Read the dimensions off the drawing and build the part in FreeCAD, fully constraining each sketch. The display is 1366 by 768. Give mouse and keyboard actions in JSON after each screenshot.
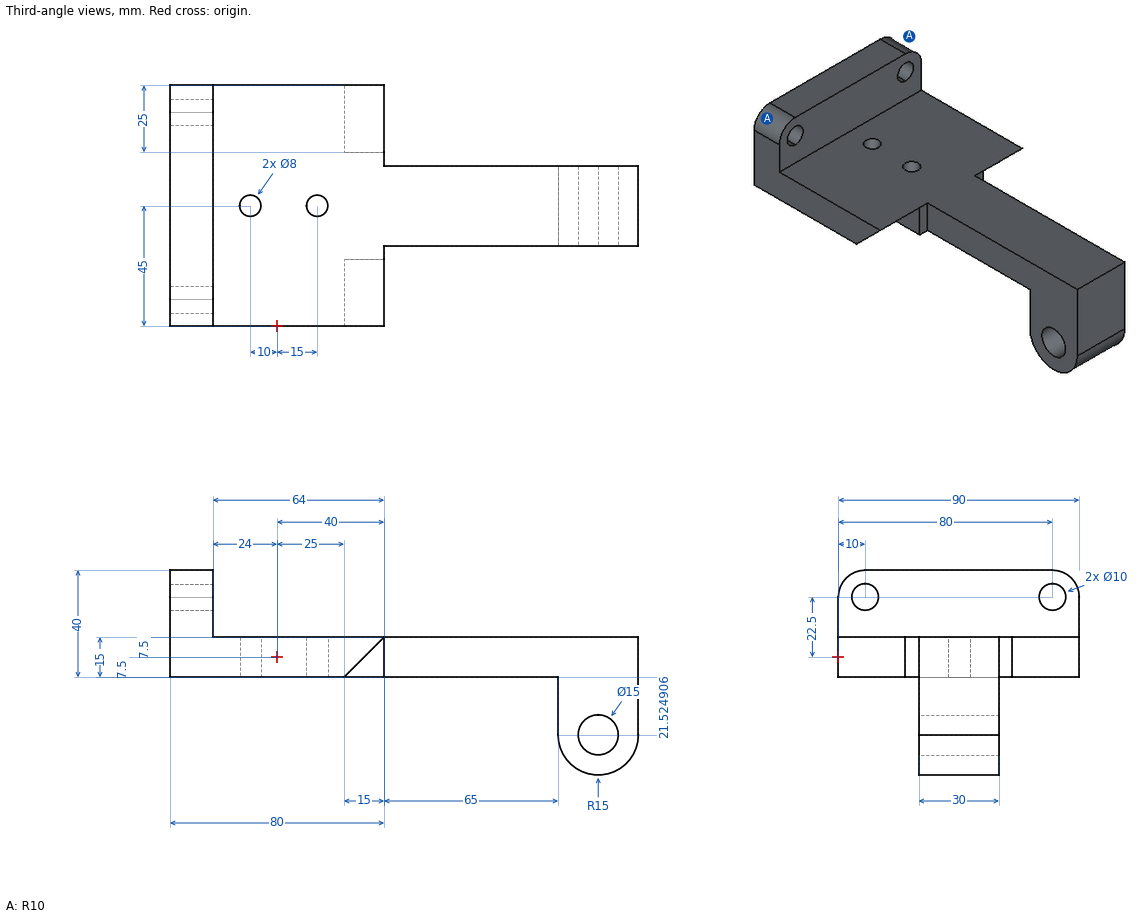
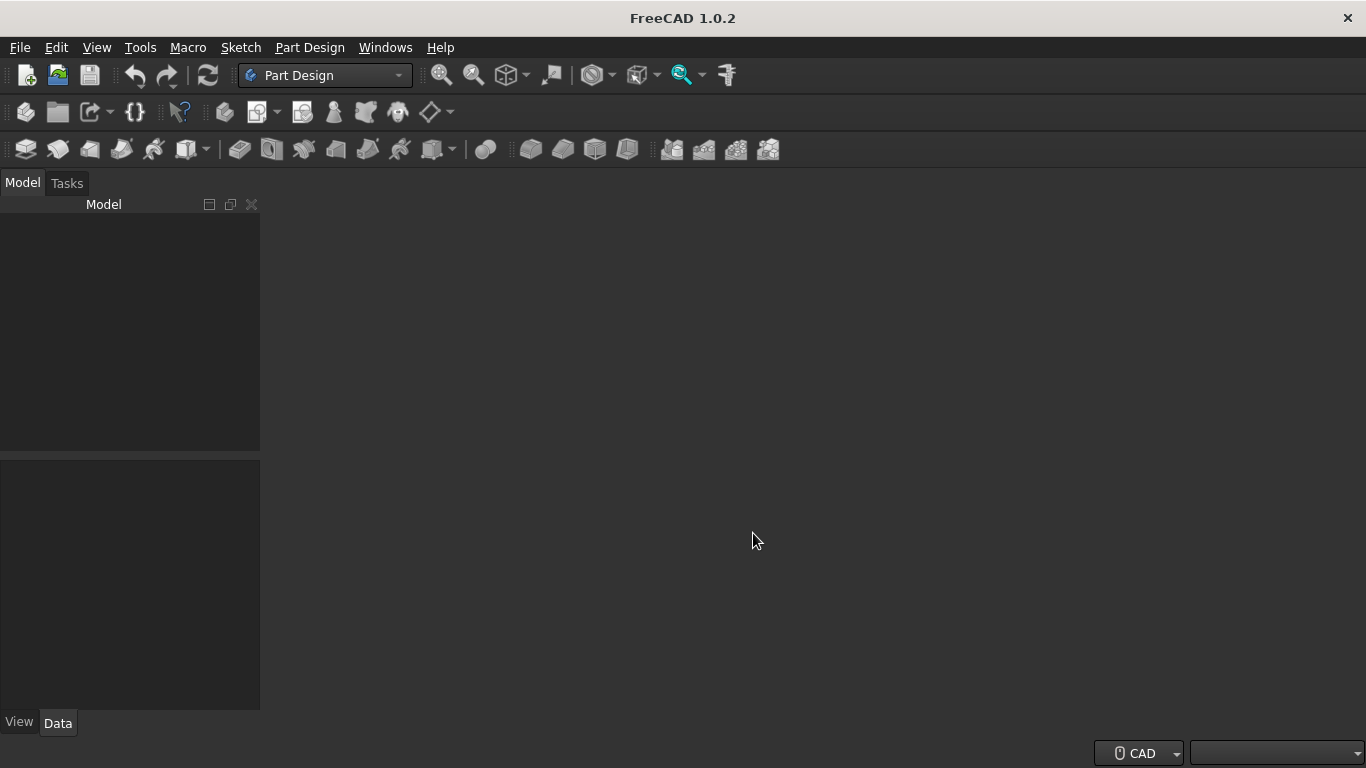
{"action": "left_click", "coordinate": [26, 76]}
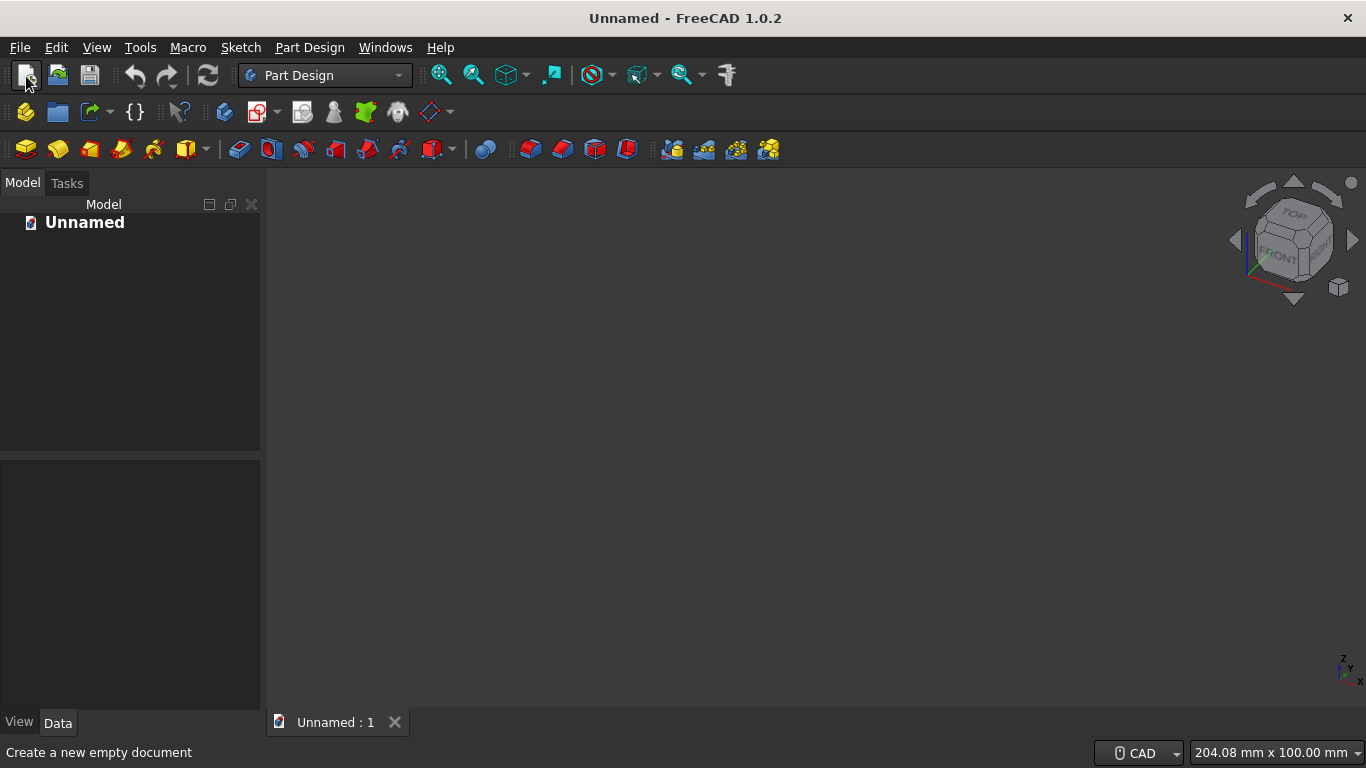
{"action": "left_click", "coordinate": [258, 112]}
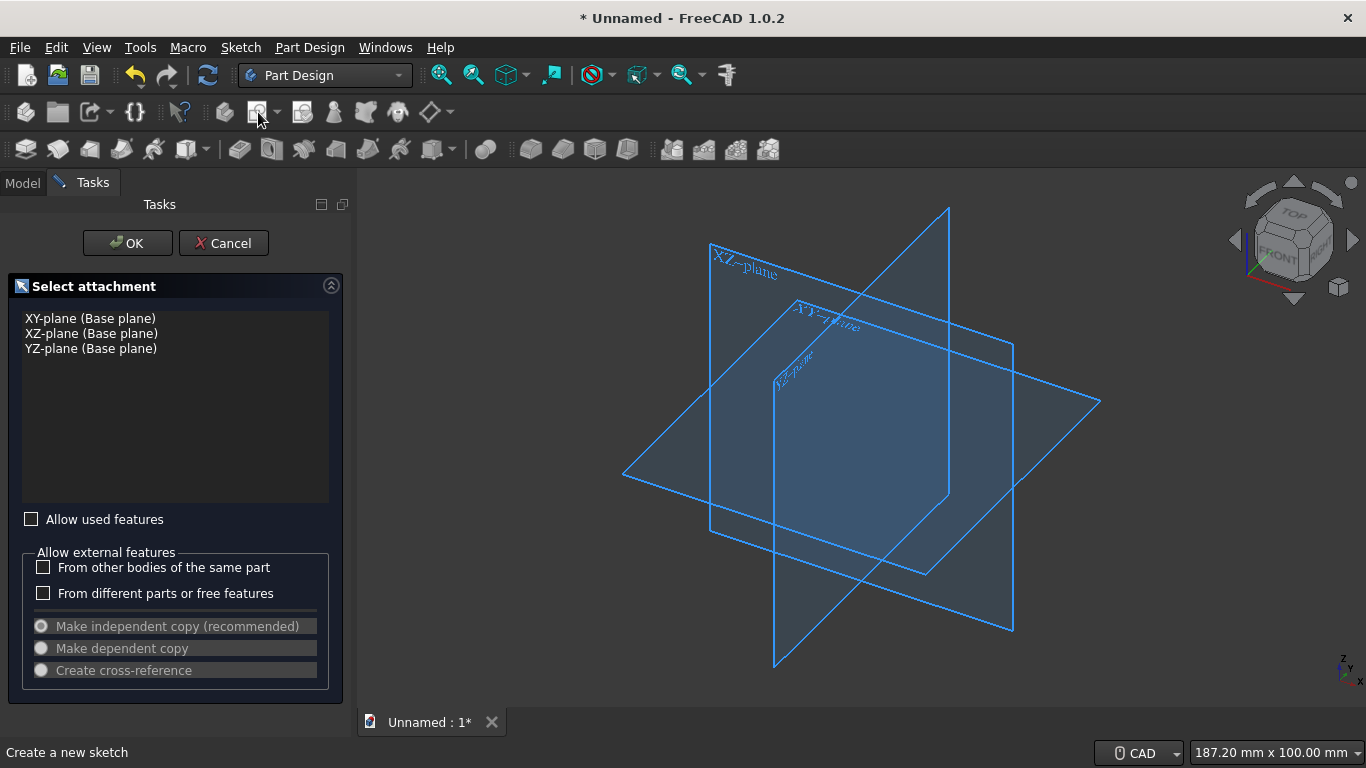
{"action": "left_click", "coordinate": [82, 334]}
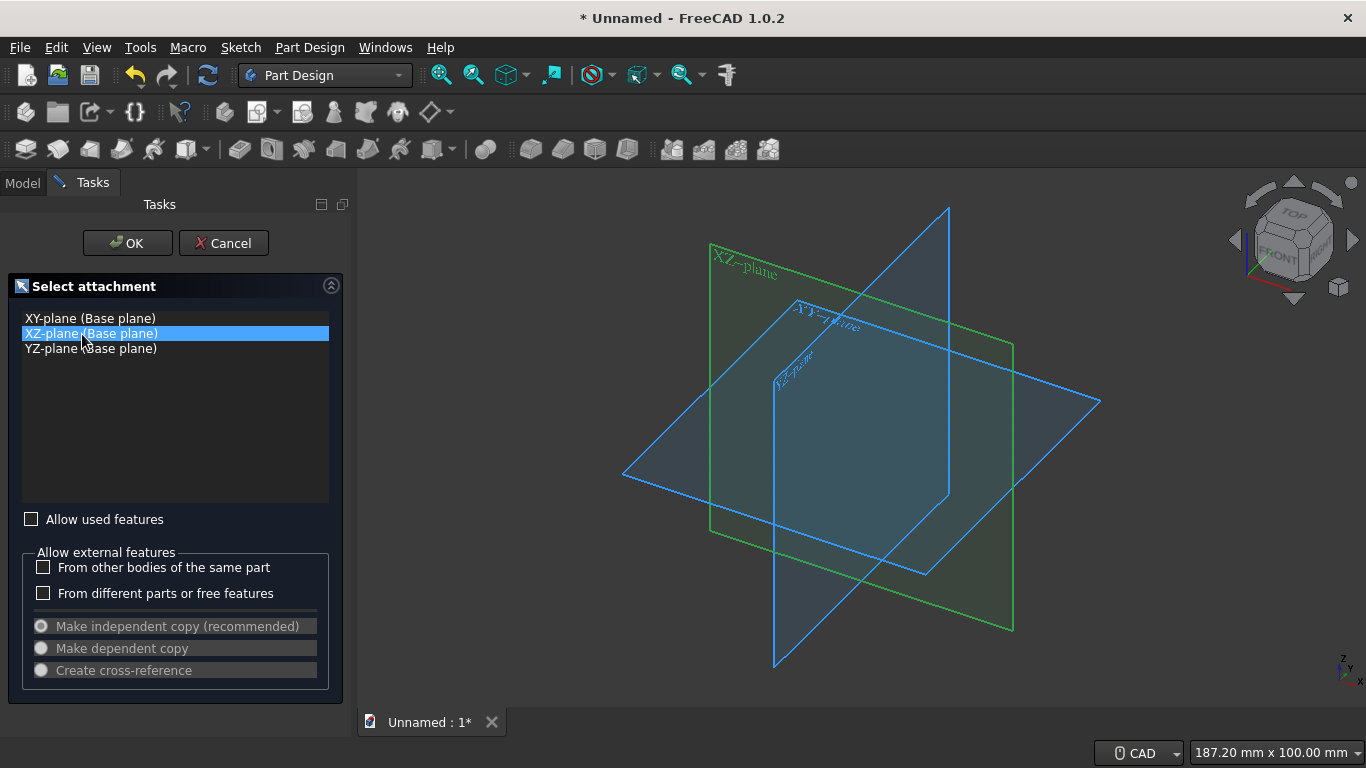
{"action": "left_click", "coordinate": [128, 243]}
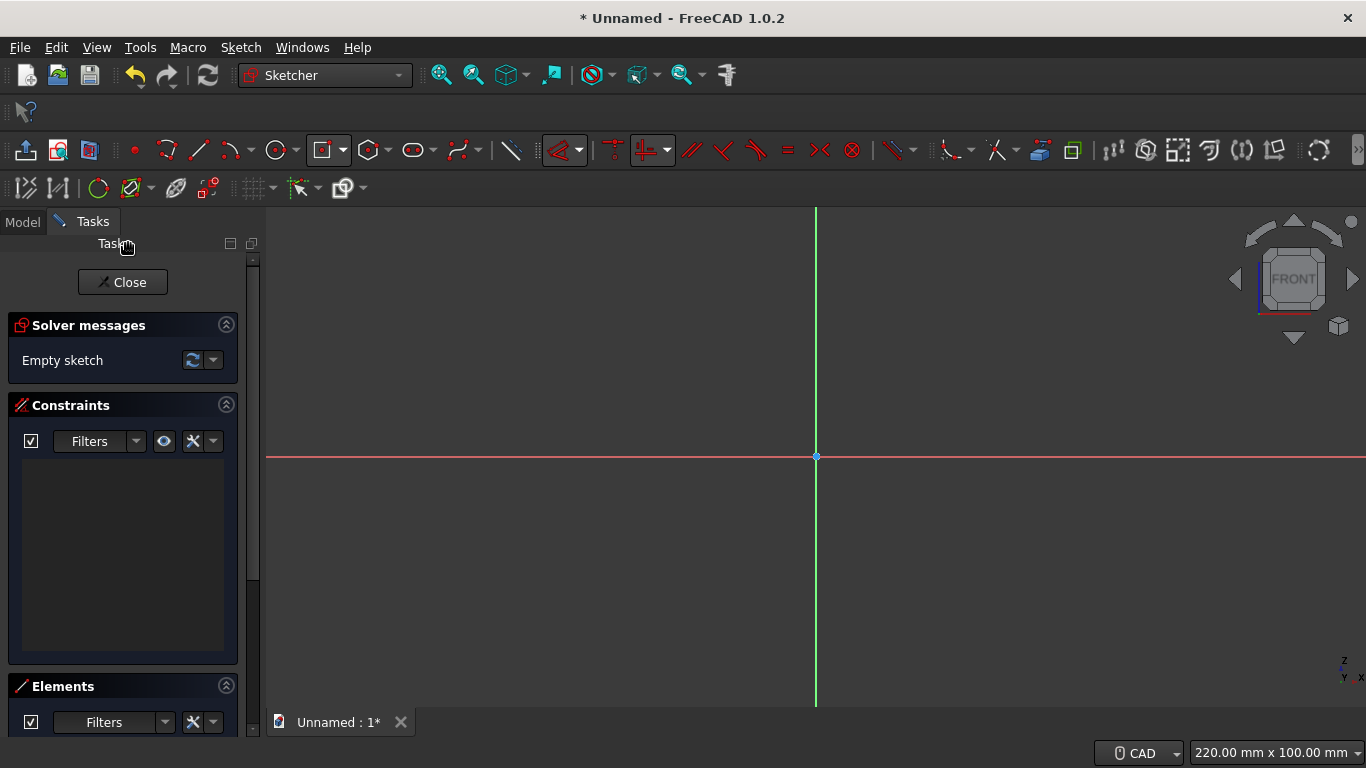
{"action": "scroll", "coordinate": [955, 267], "scroll_direction": "up", "scroll_amount": 2}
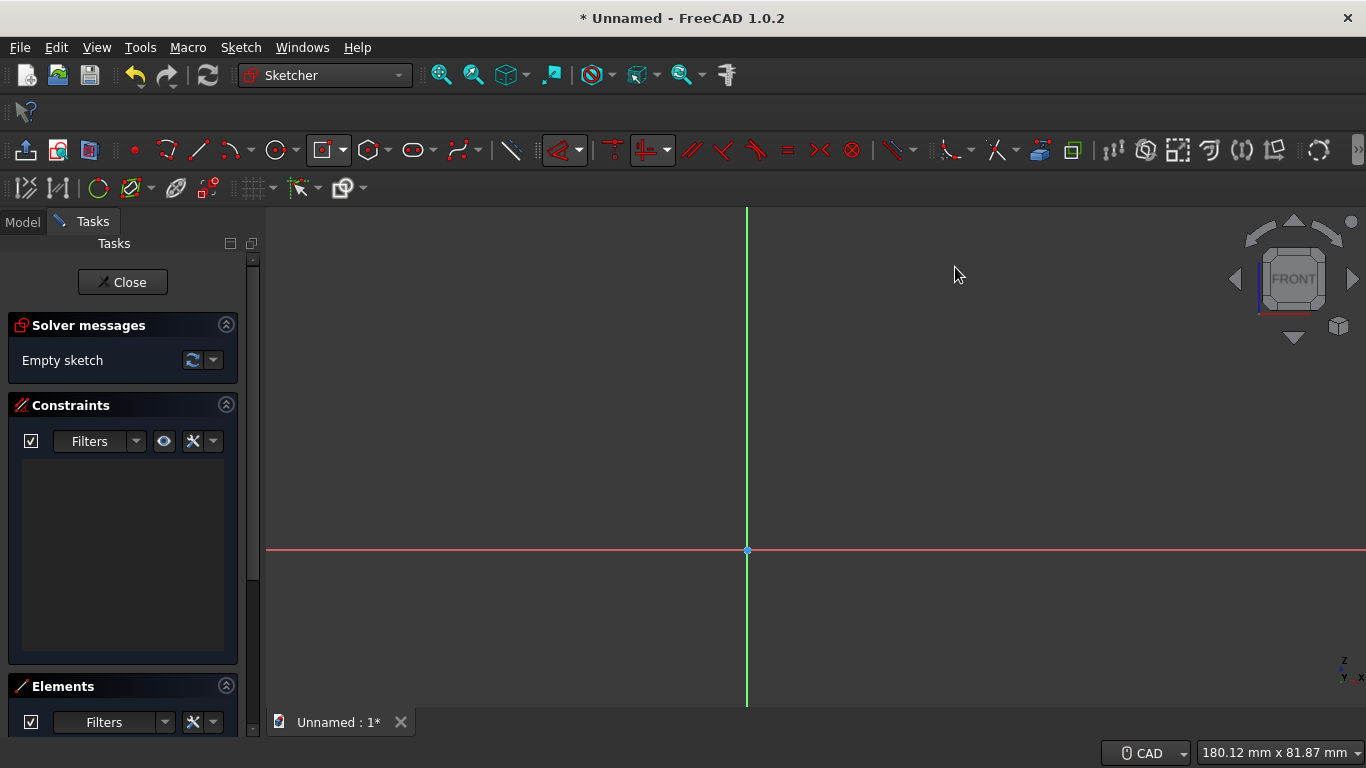
{"action": "left_click", "coordinate": [168, 150]}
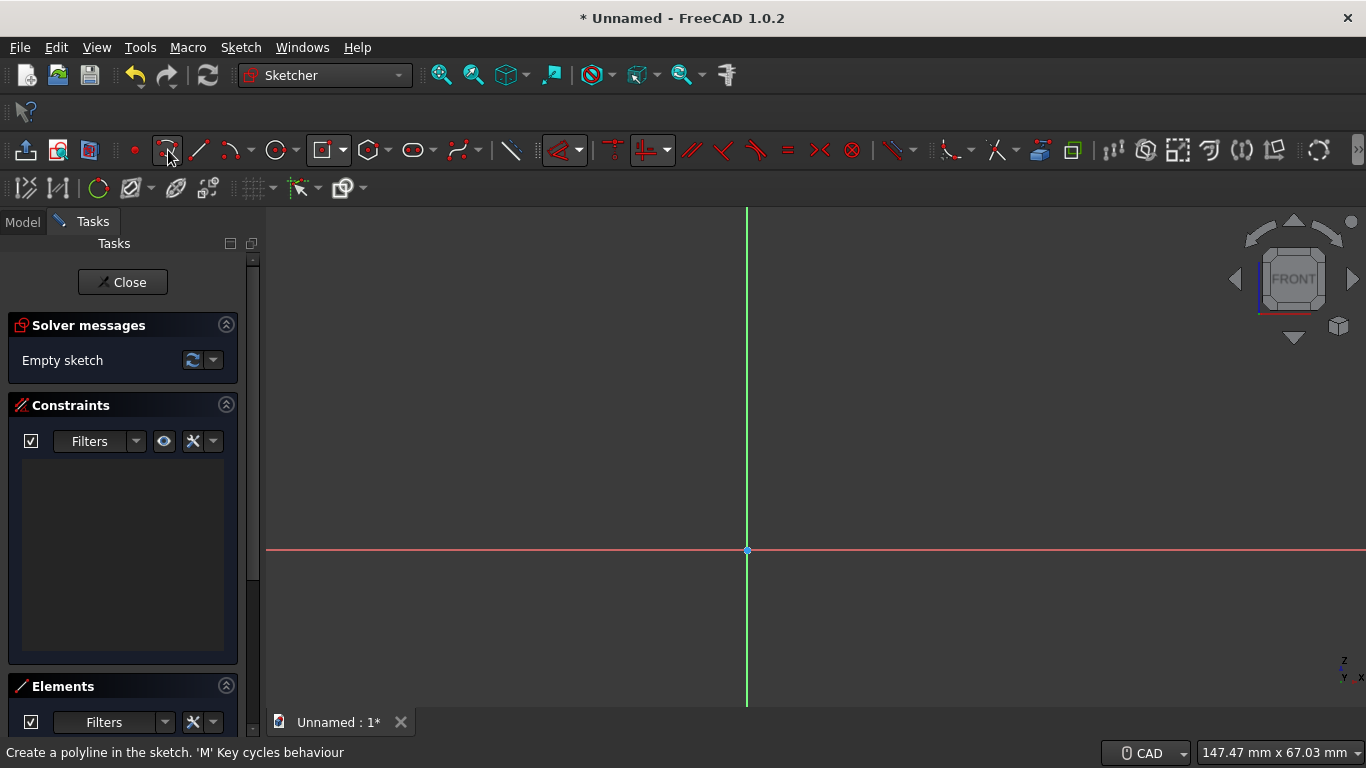
{"action": "left_click", "coordinate": [568, 494]}
{"action": "left_click", "coordinate": [1046, 494]}
{"action": "left_click", "coordinate": [1046, 606]}
{"action": "left_click", "coordinate": [449, 606]}
{"action": "left_click", "coordinate": [449, 308]}
{"action": "left_click", "coordinate": [568, 308]}
{"action": "left_click", "coordinate": [568, 495]}
{"action": "key", "text": "Escape"}
{"action": "key", "text": "Escape"}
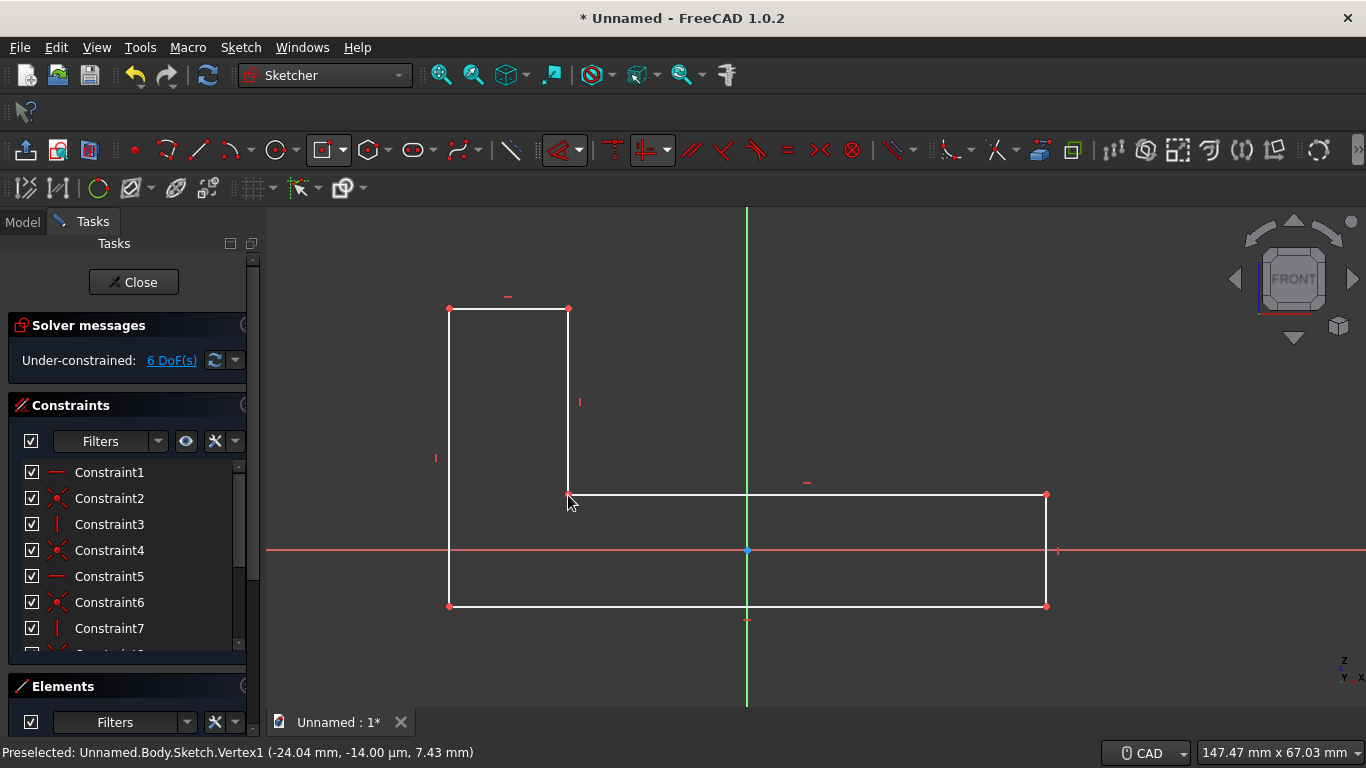
{"action": "left_click", "coordinate": [558, 150]}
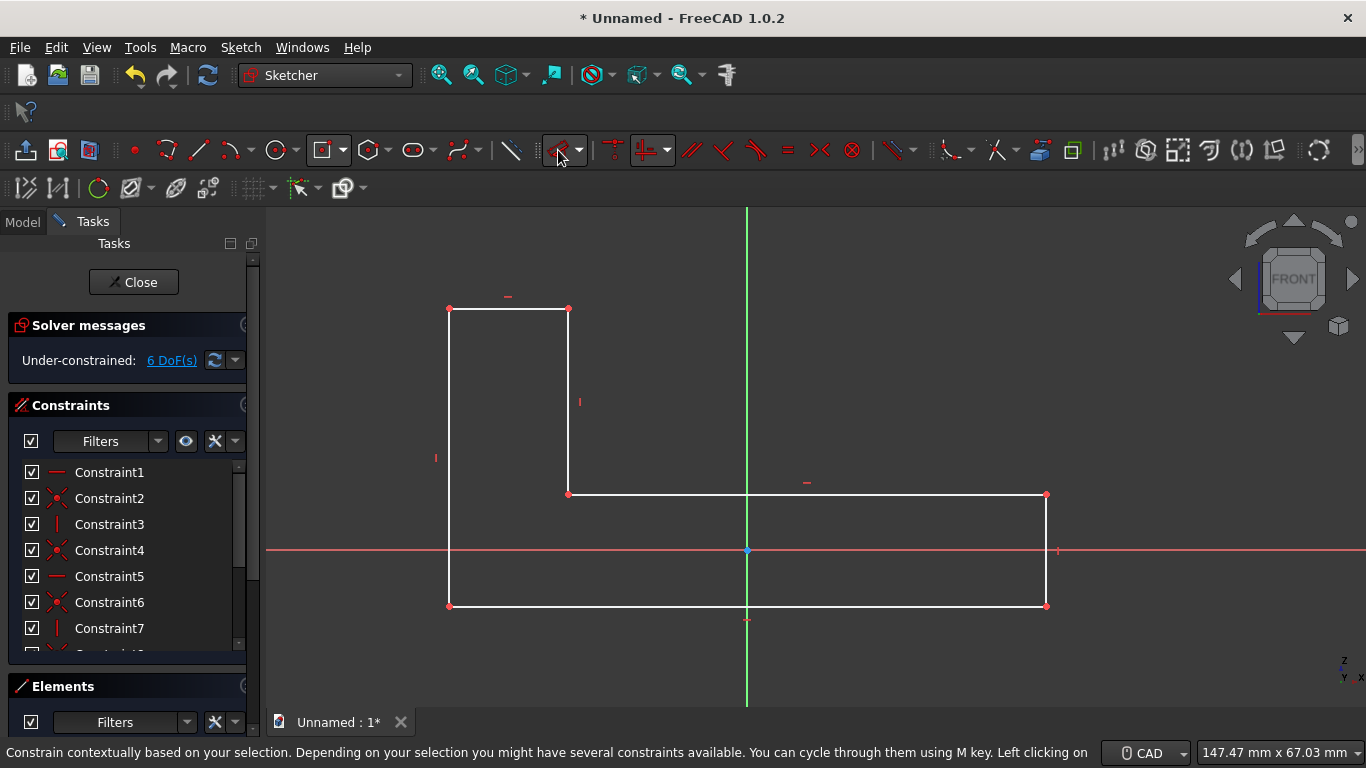
{"action": "left_click", "coordinate": [711, 495]}
{"action": "left_click", "coordinate": [807, 529]}